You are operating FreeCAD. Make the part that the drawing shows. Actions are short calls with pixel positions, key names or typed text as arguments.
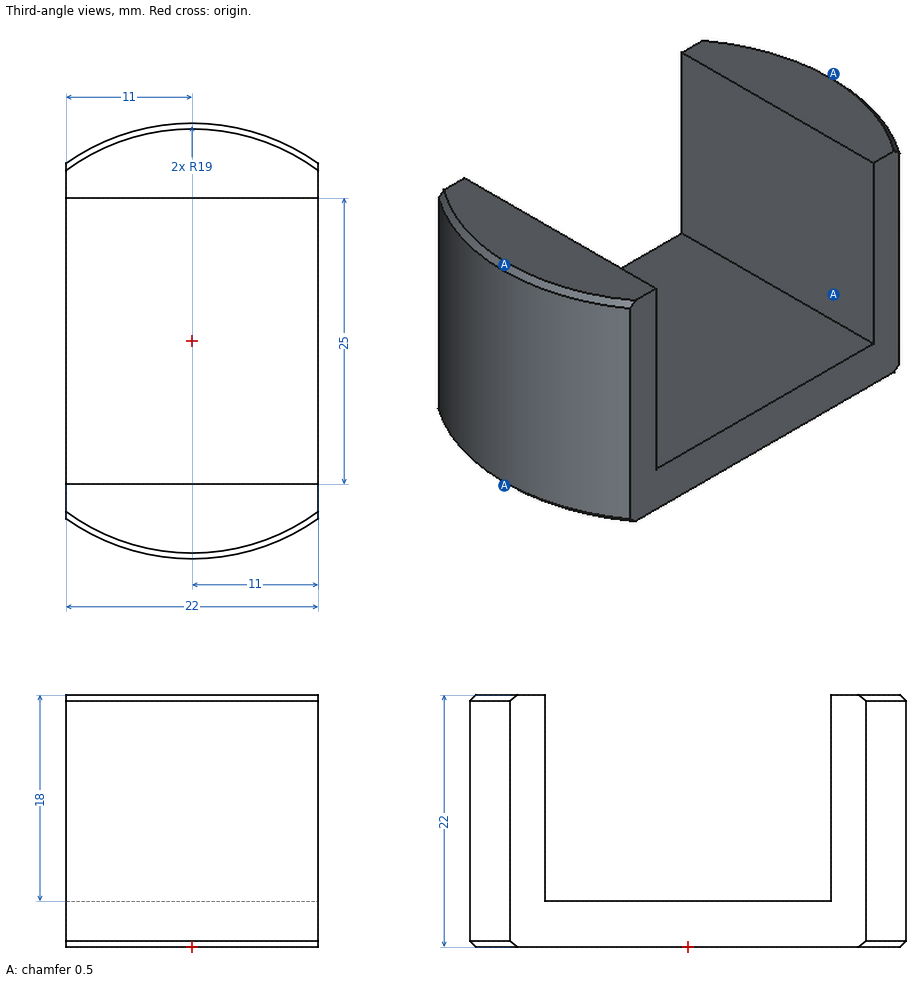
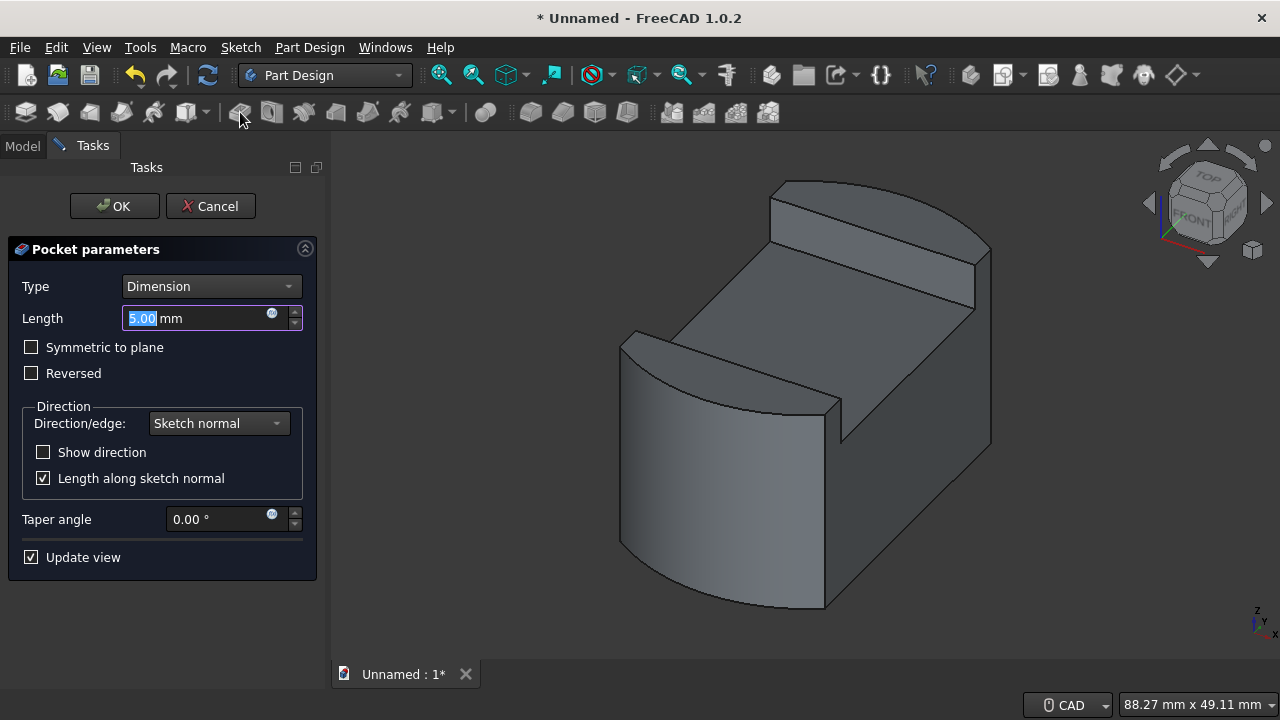
text(18)
key(Tab)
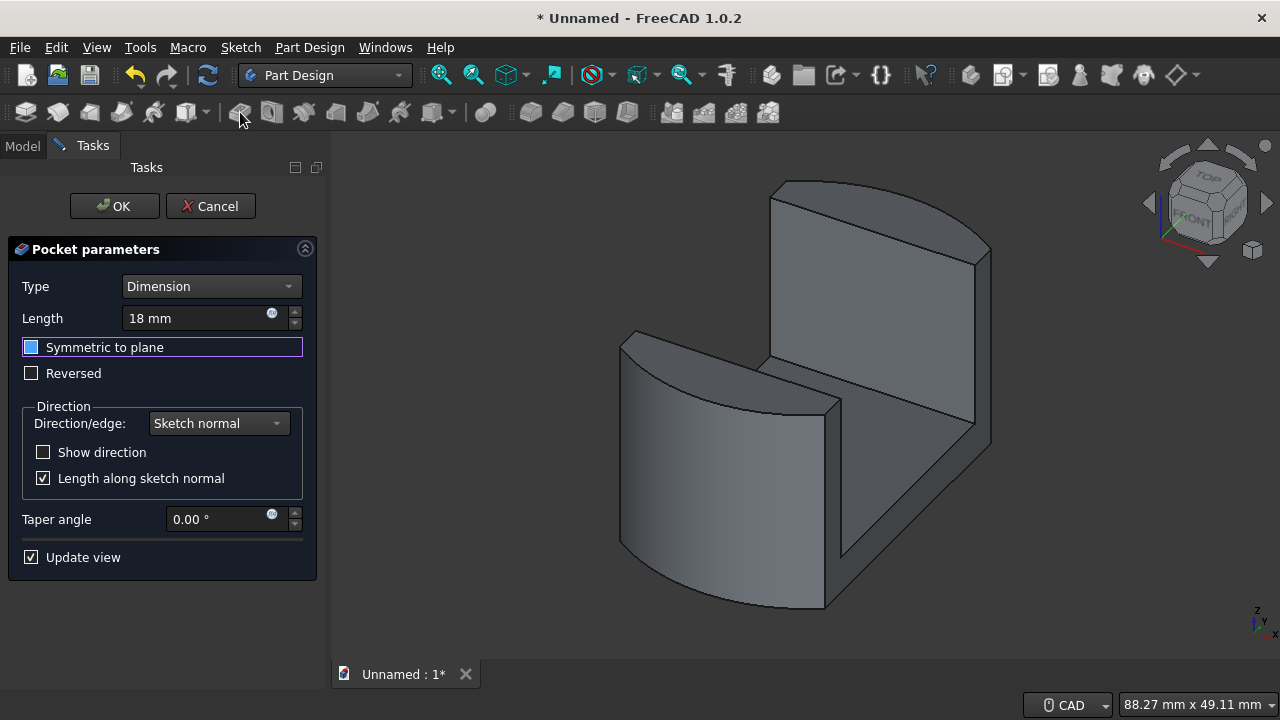
click(115, 206)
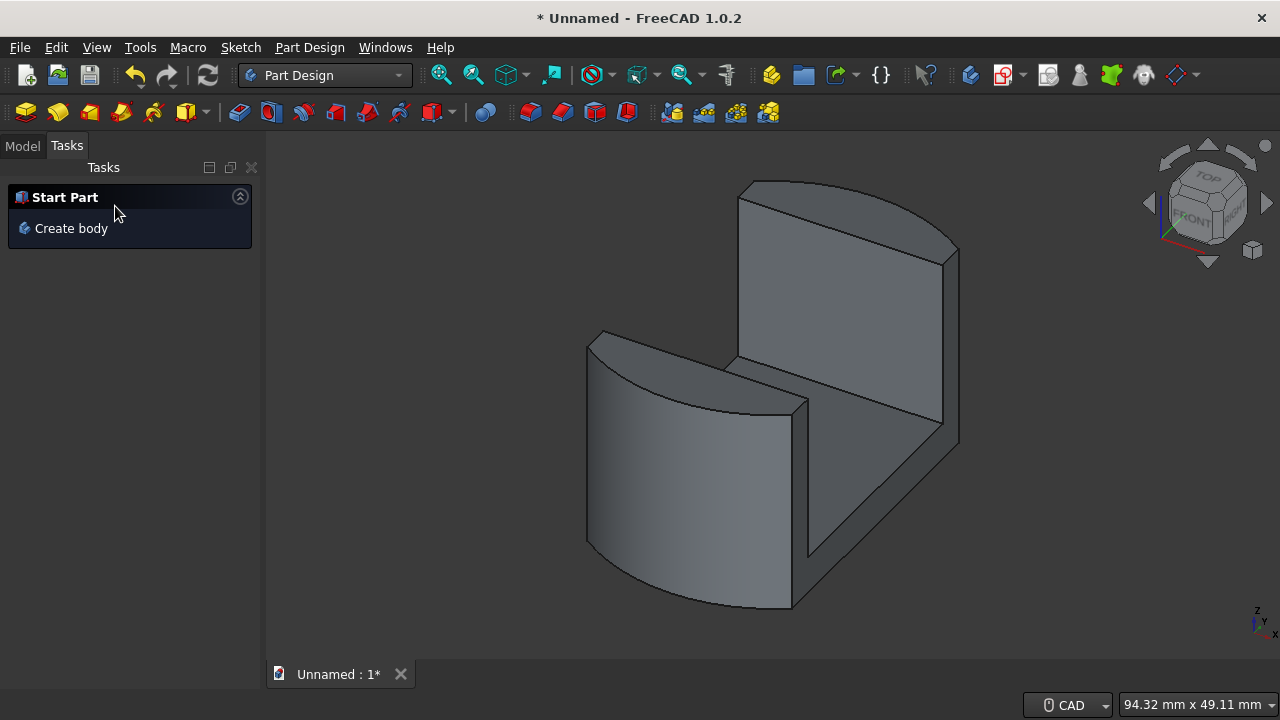
click(853, 189)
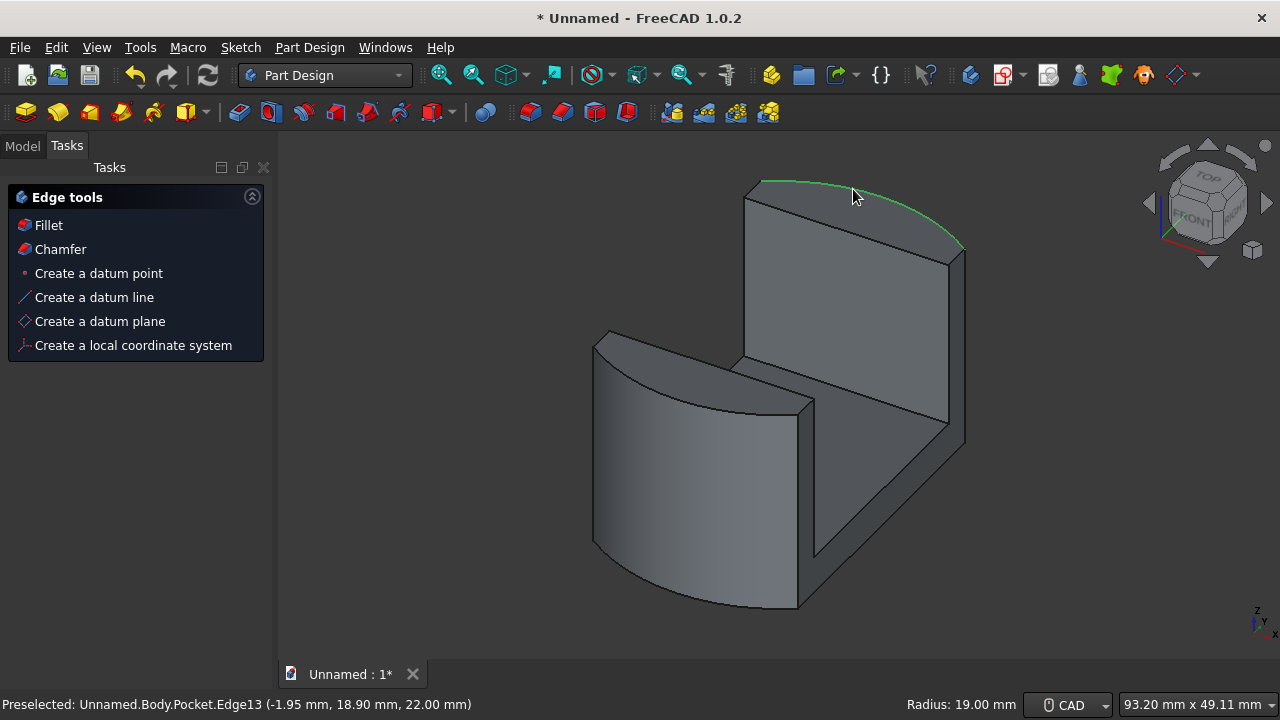
click(677, 399, ctrl)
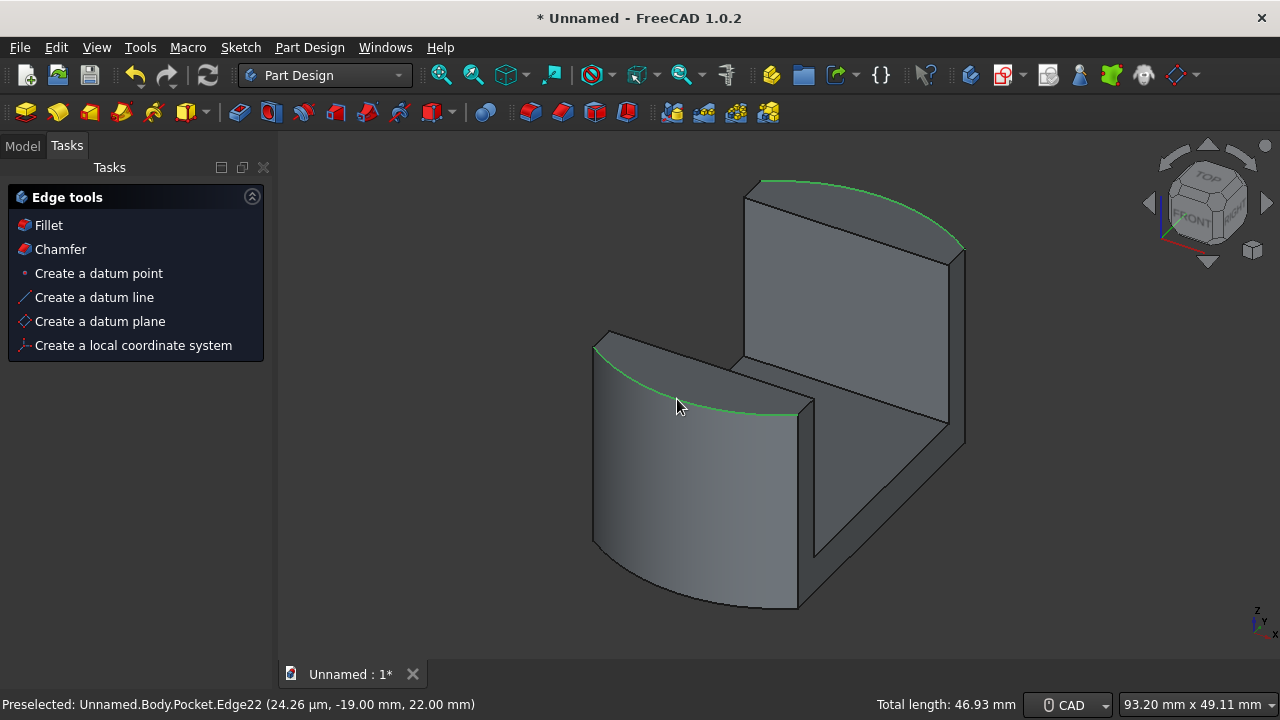
key(0)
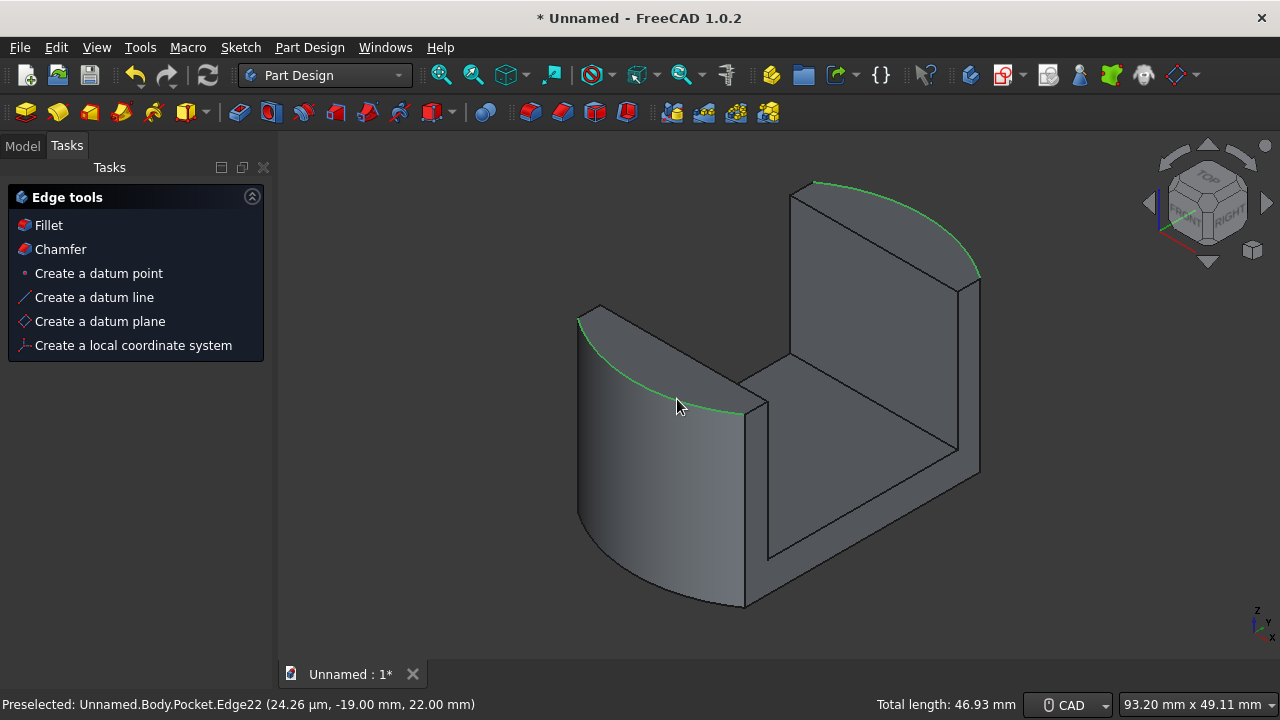
key(2)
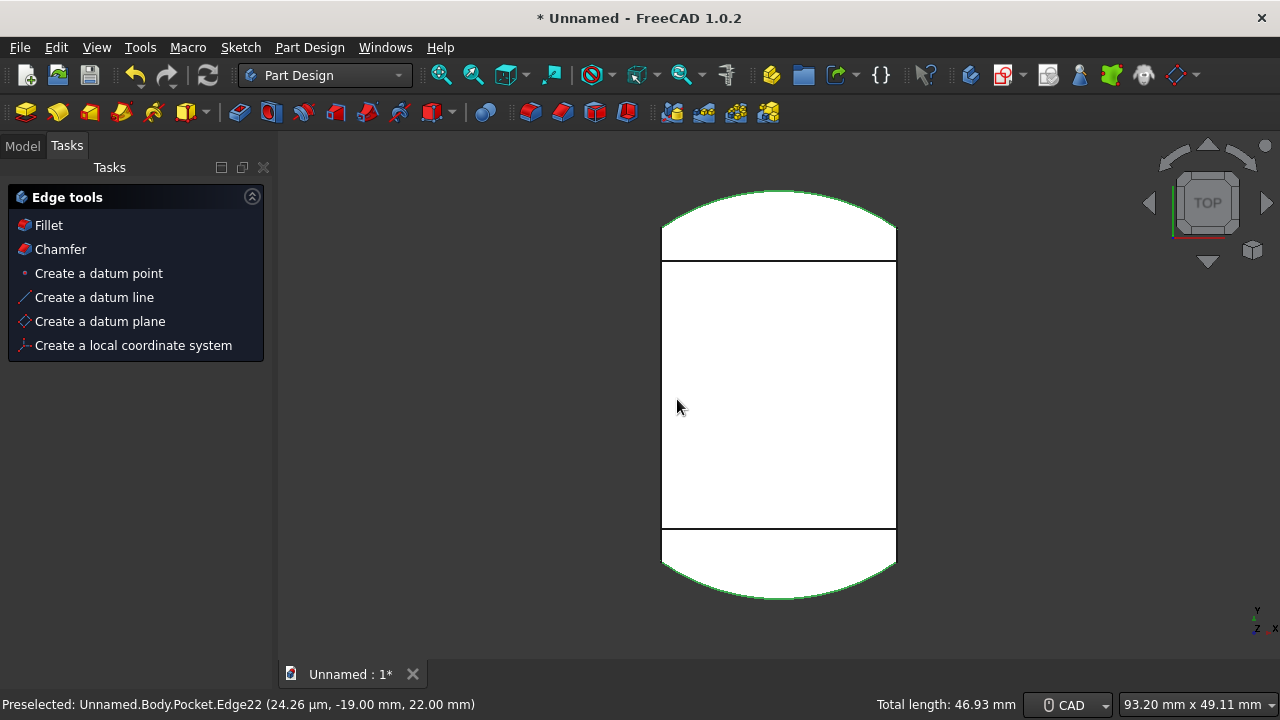
key(1)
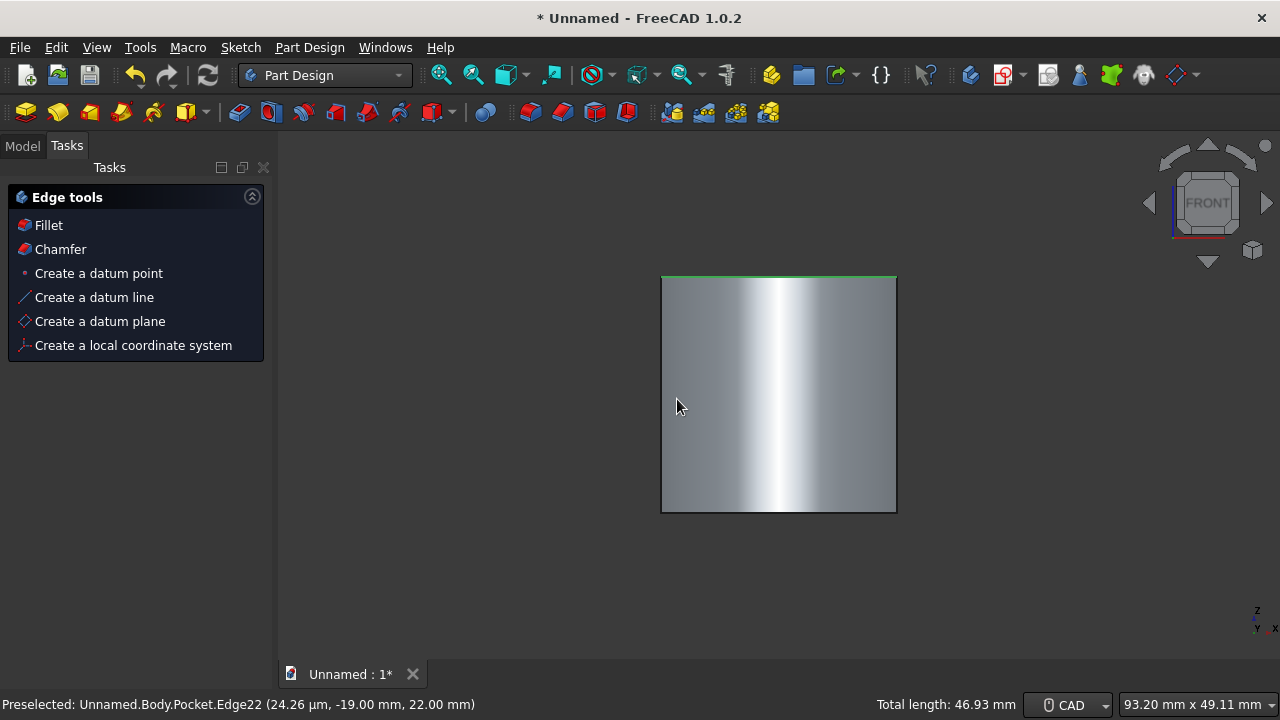
click(442, 76)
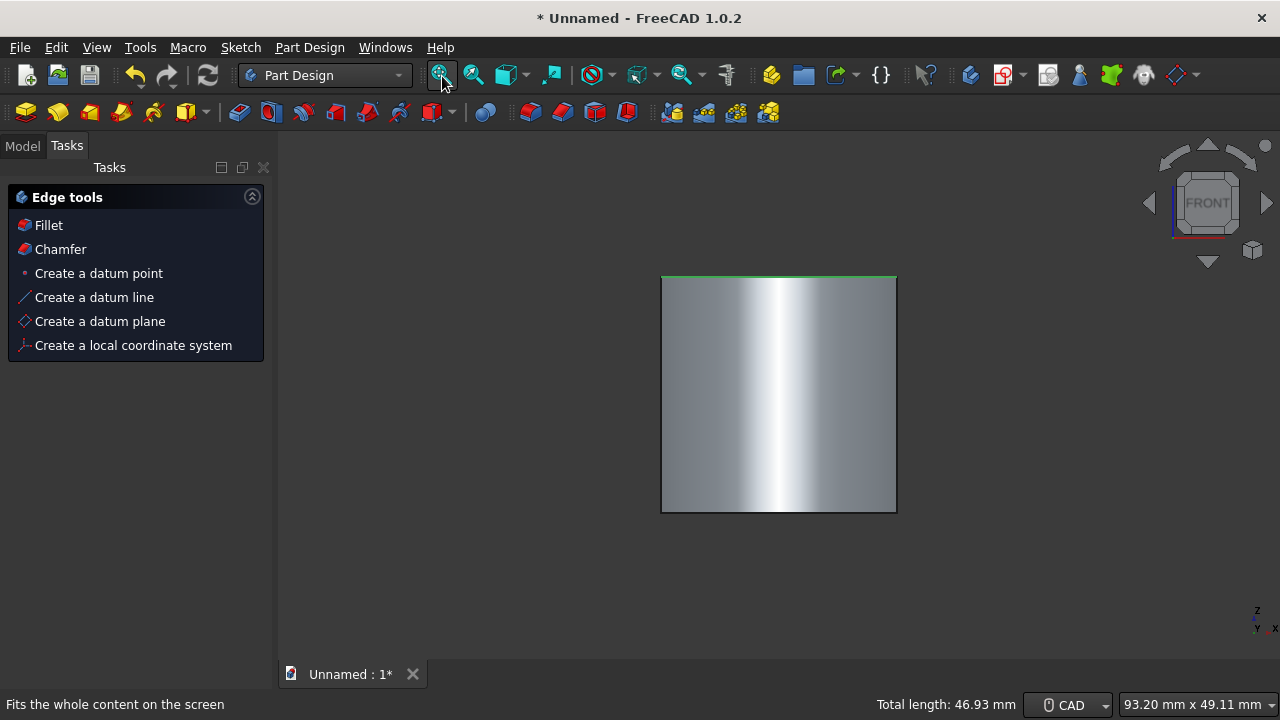
click(779, 512, ctrl)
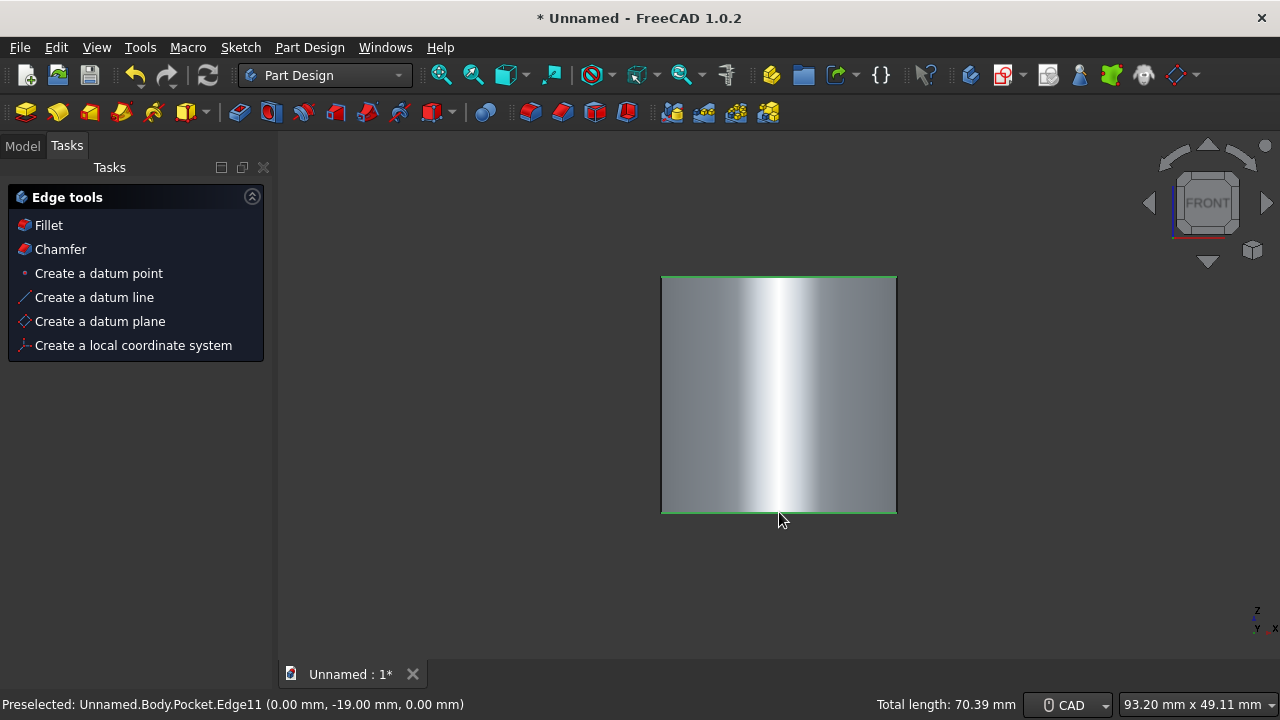
key(3)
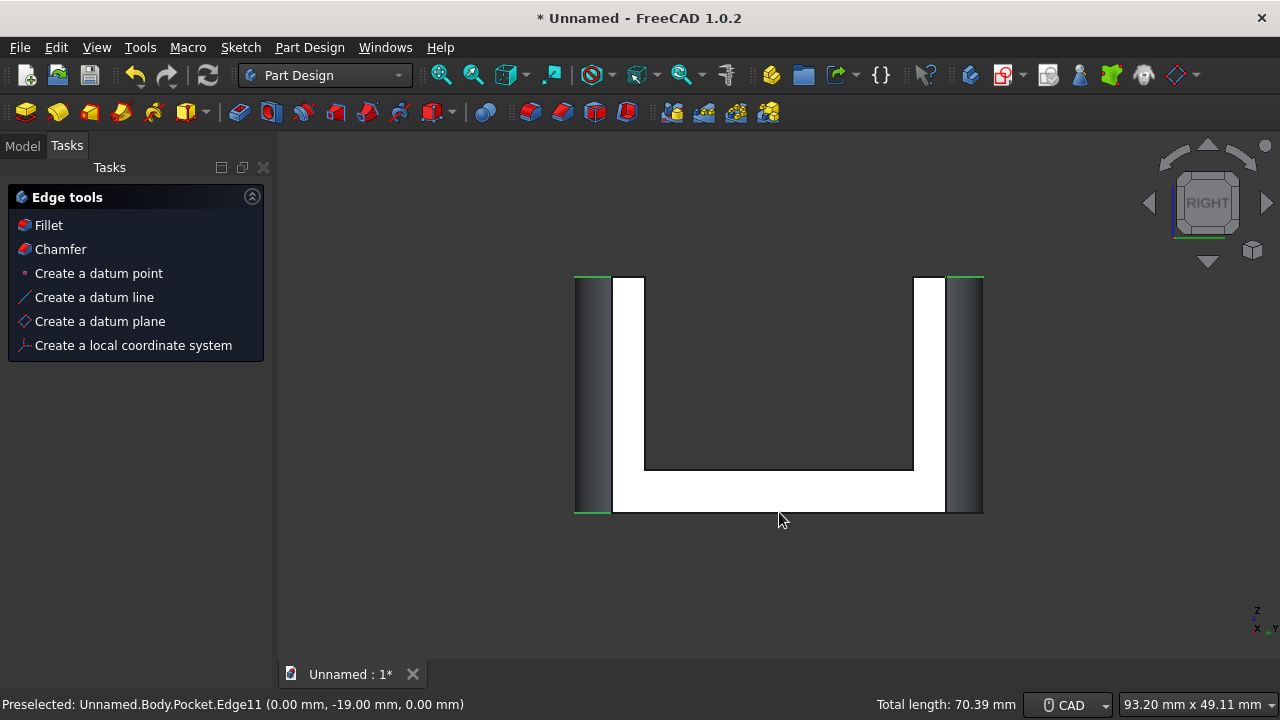
click(442, 76)